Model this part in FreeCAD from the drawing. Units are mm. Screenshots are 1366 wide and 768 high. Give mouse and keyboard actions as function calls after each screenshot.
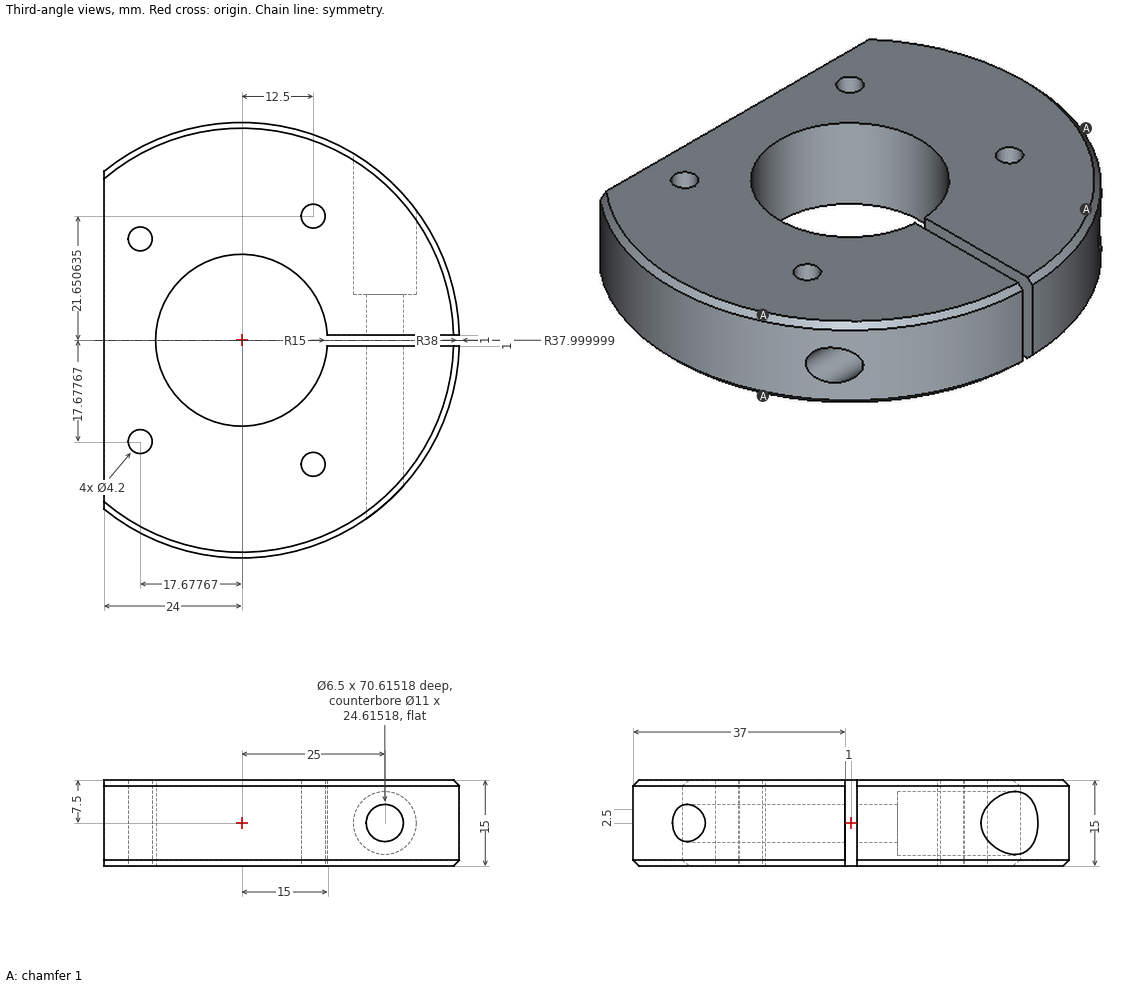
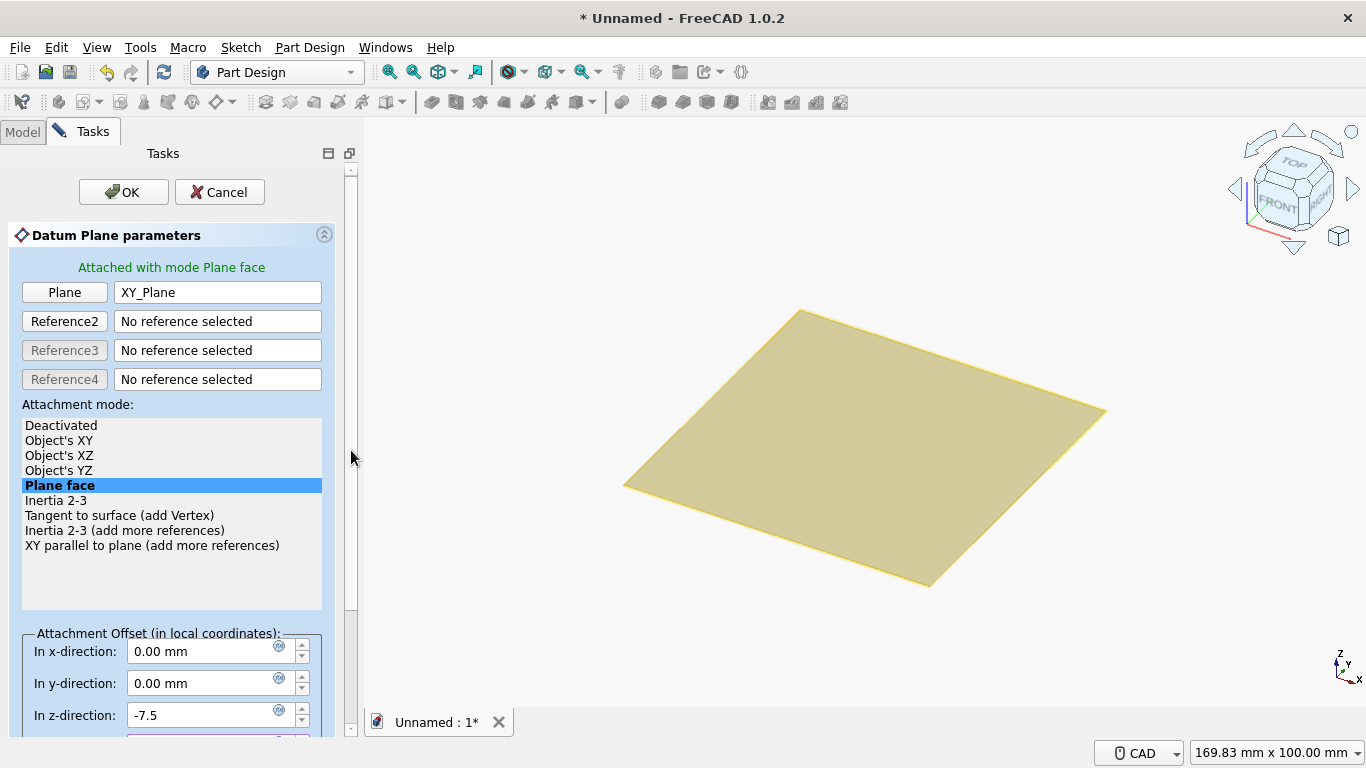
click(124, 192)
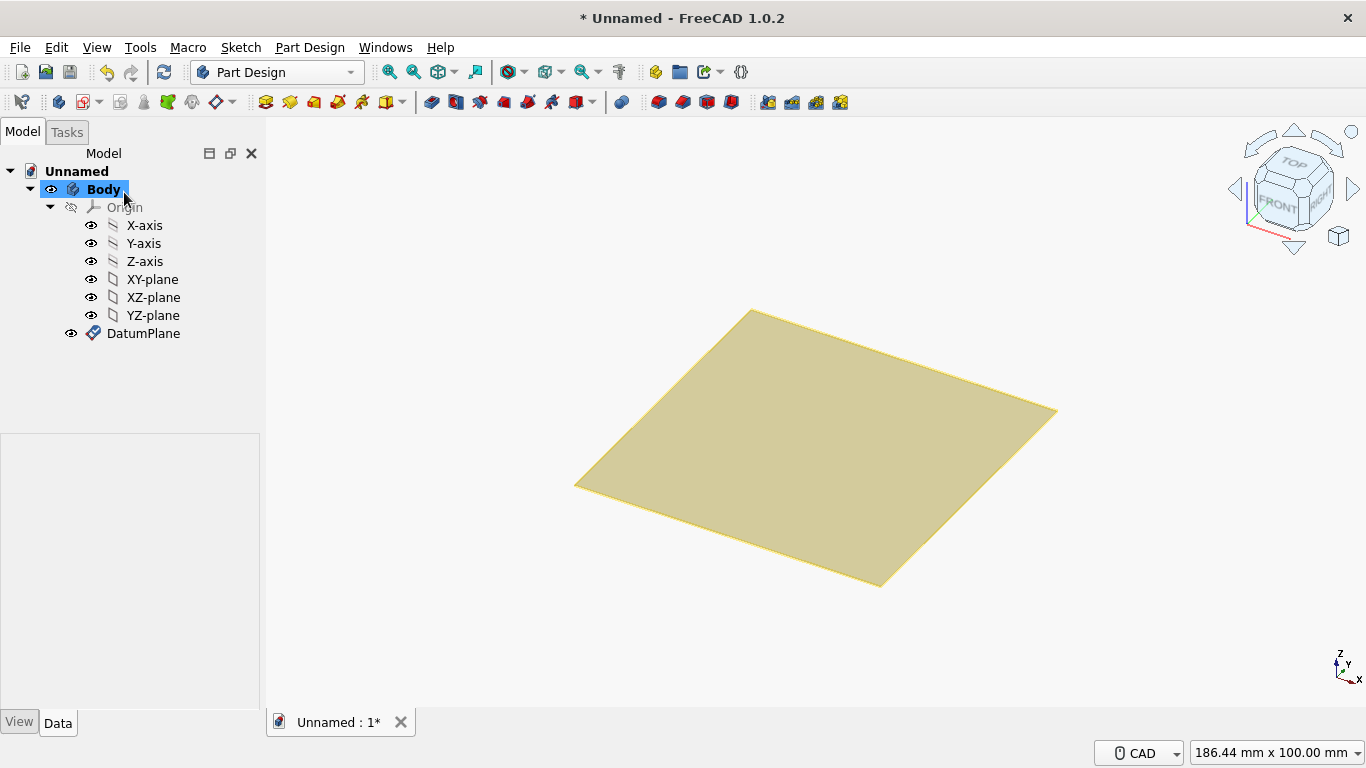
click(116, 333)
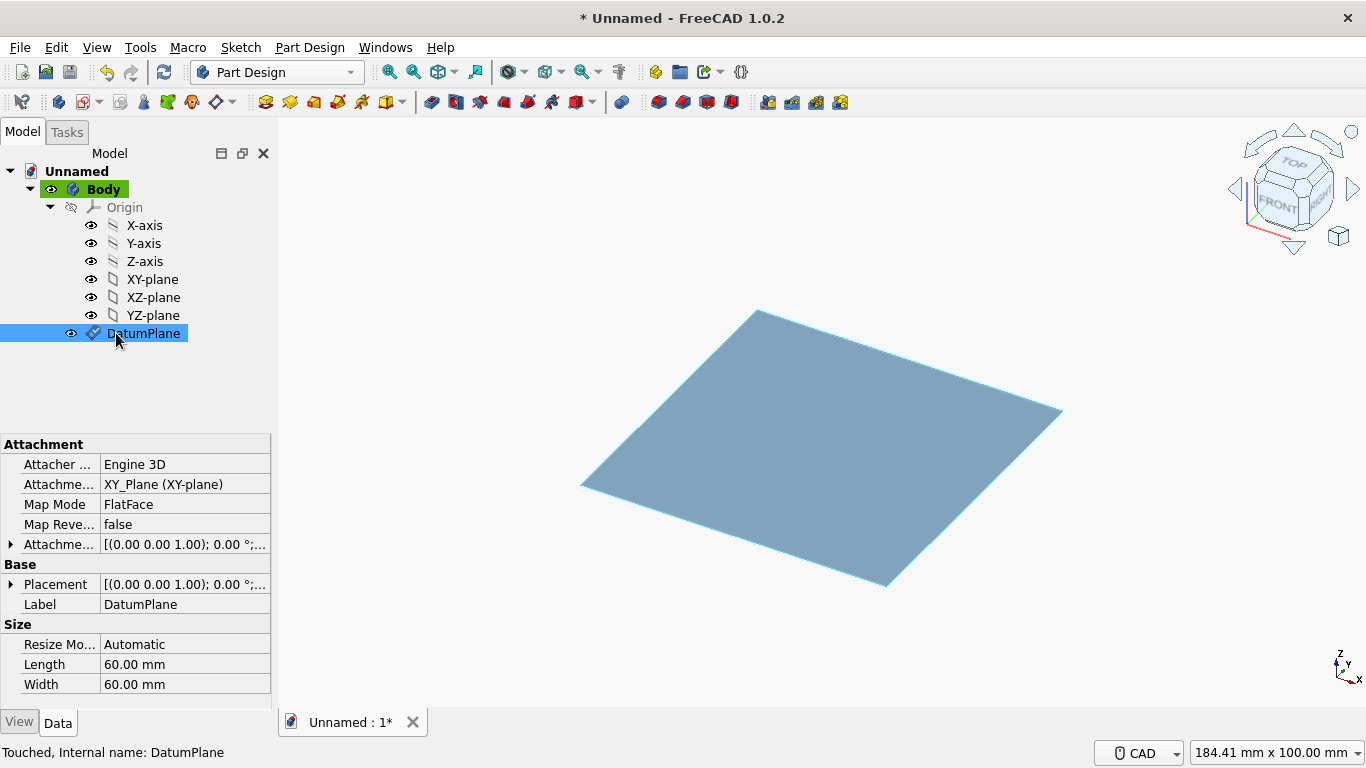
click(84, 102)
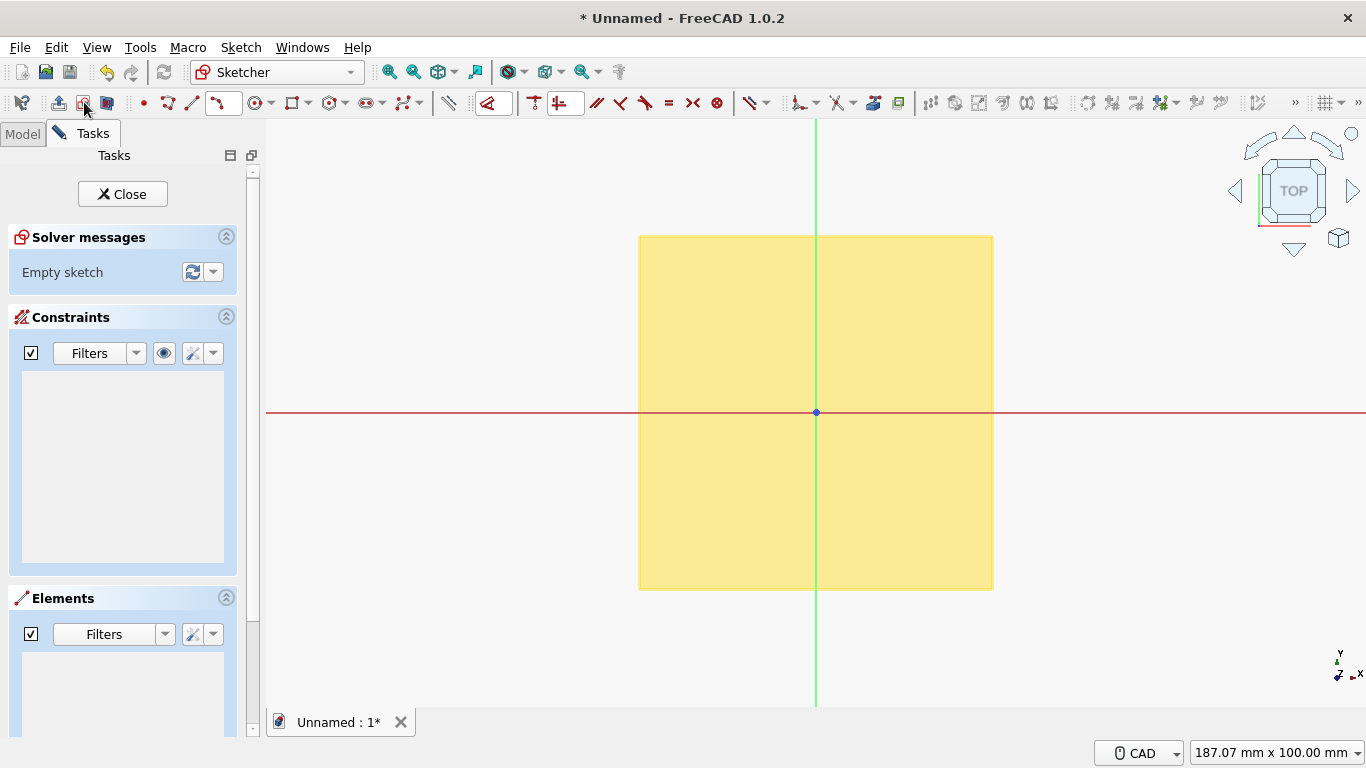
click(192, 104)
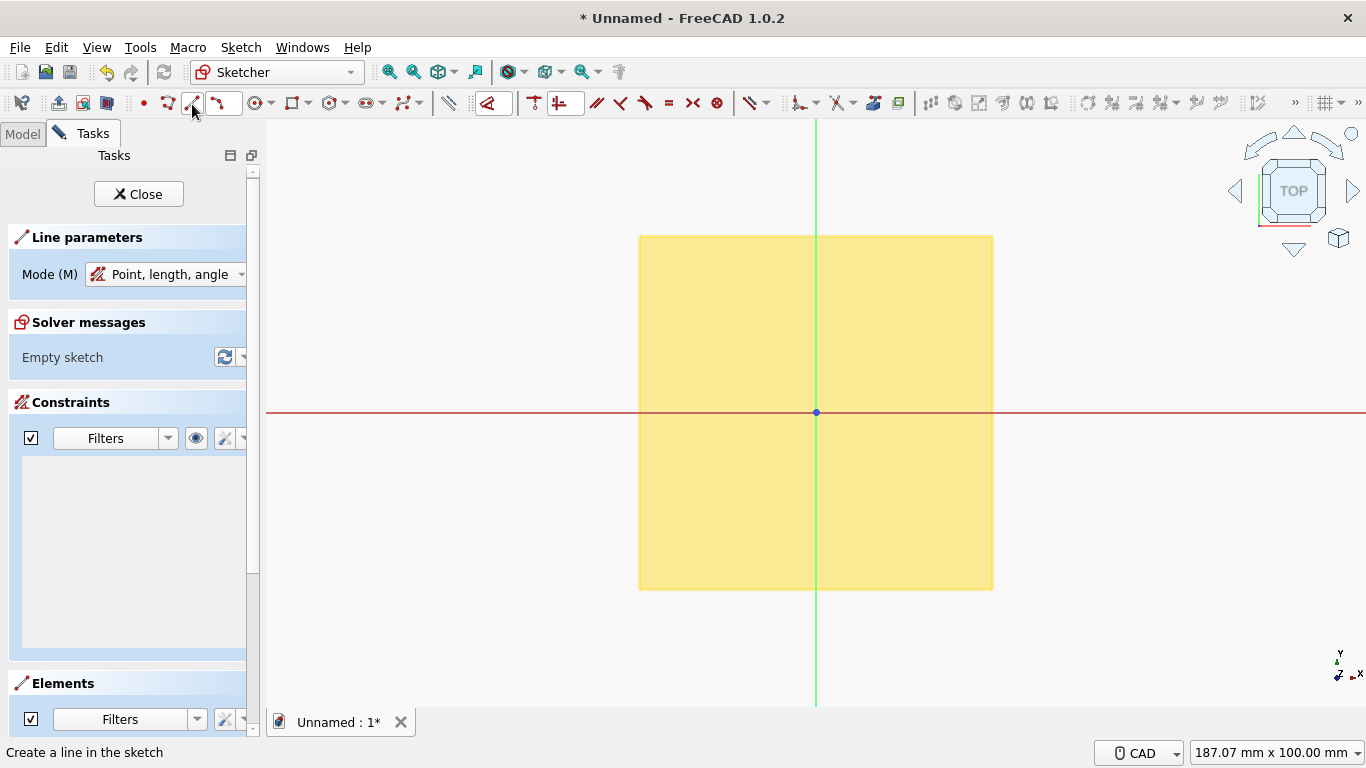
click(675, 586)
click(675, 240)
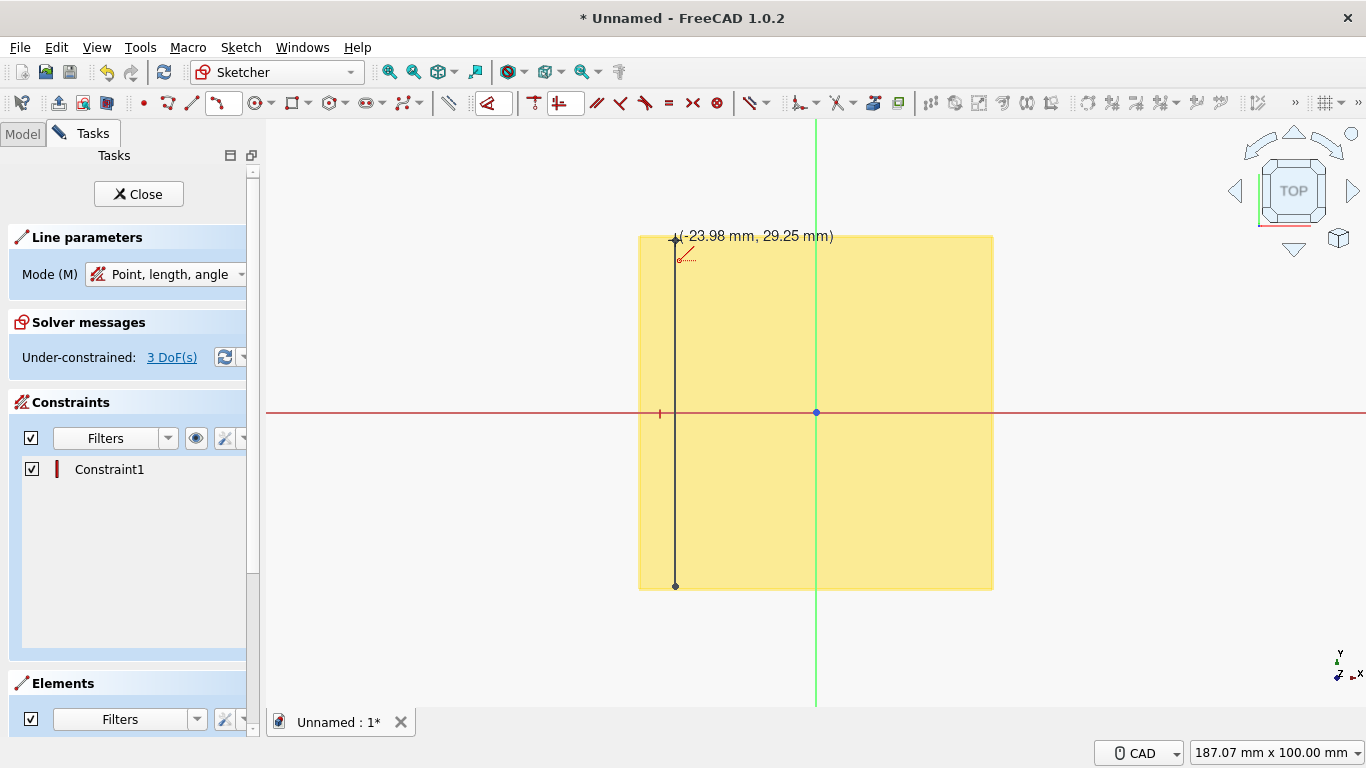
click(218, 104)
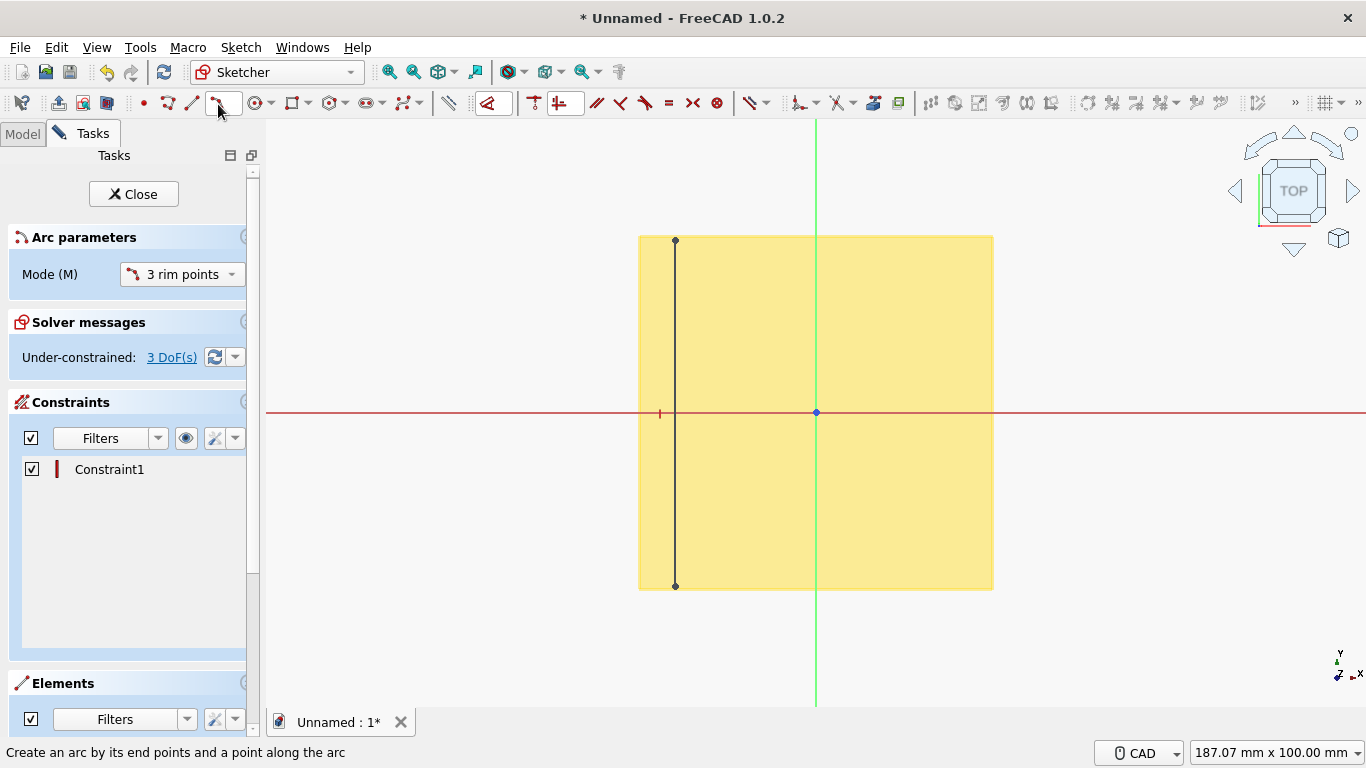
click(675, 241)
click(675, 587)
click(1017, 510)
key(Escape)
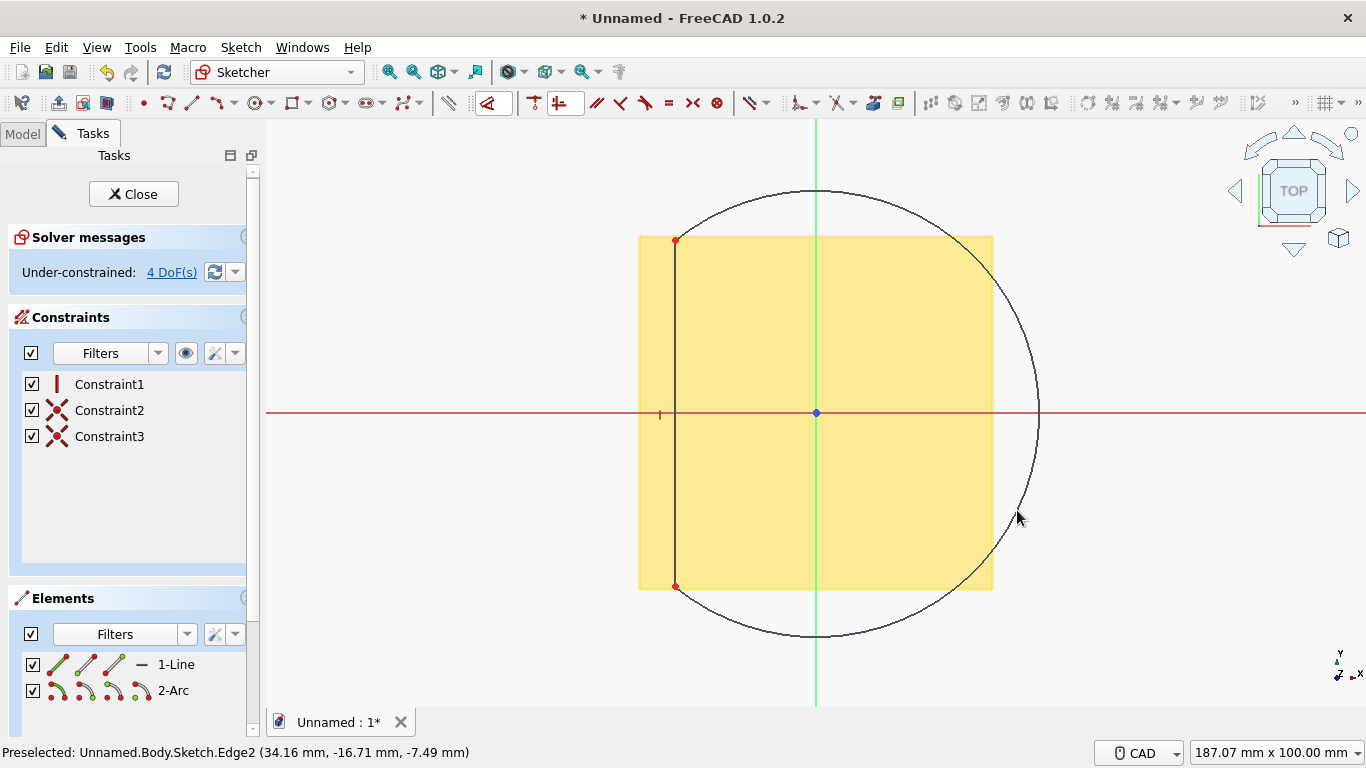
drag(806, 403, 826, 424)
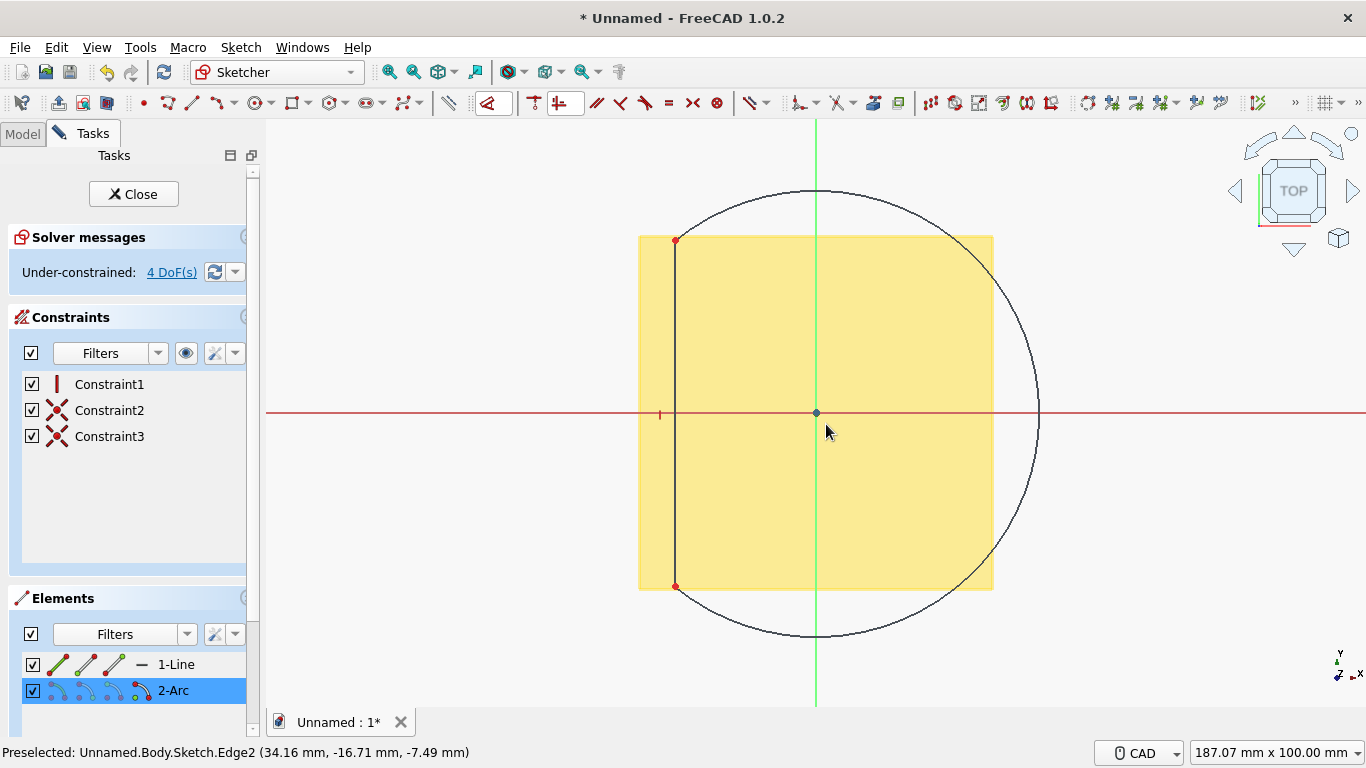
click(534, 104)